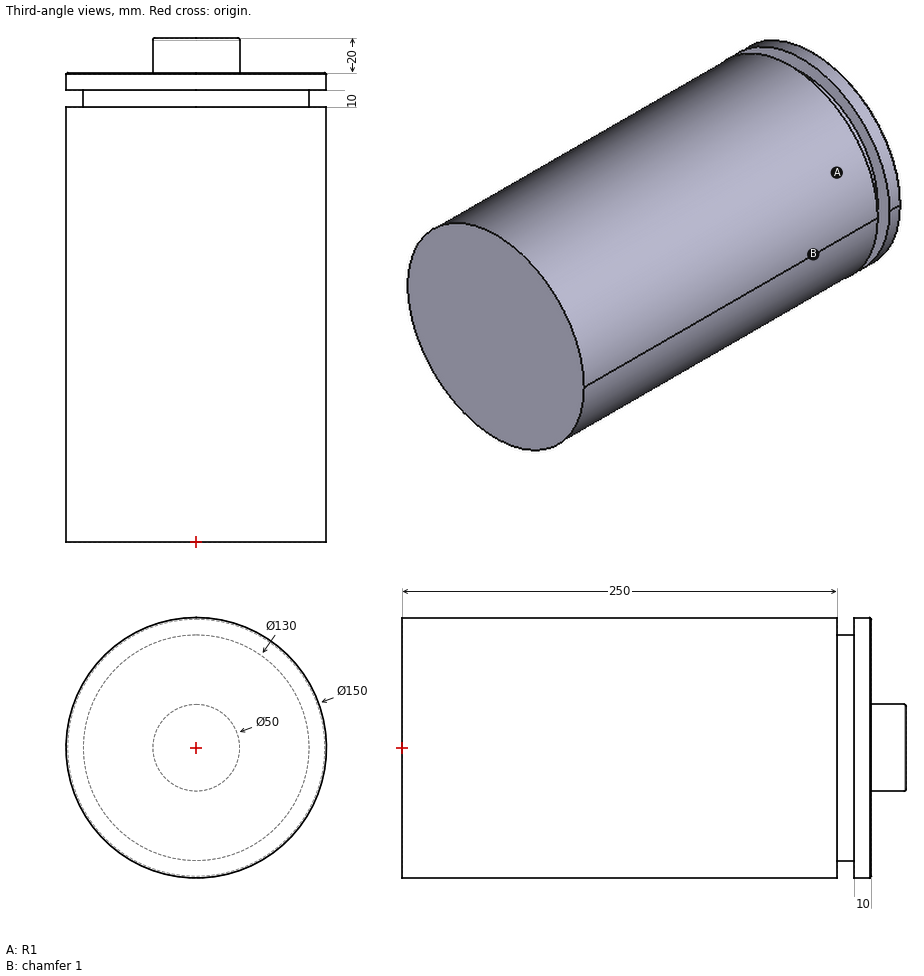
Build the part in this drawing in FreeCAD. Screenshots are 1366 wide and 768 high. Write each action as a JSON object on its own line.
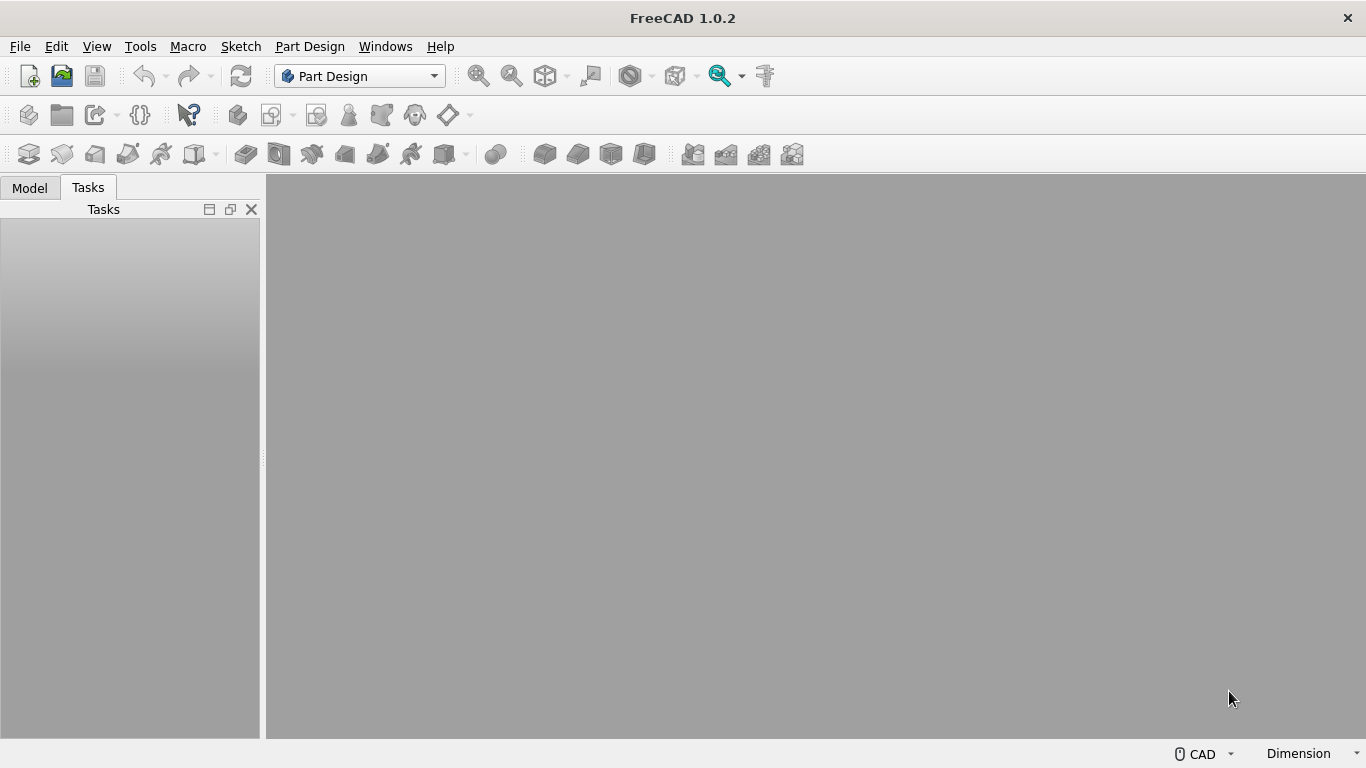
{"action": "key", "text": "ctrl+n"}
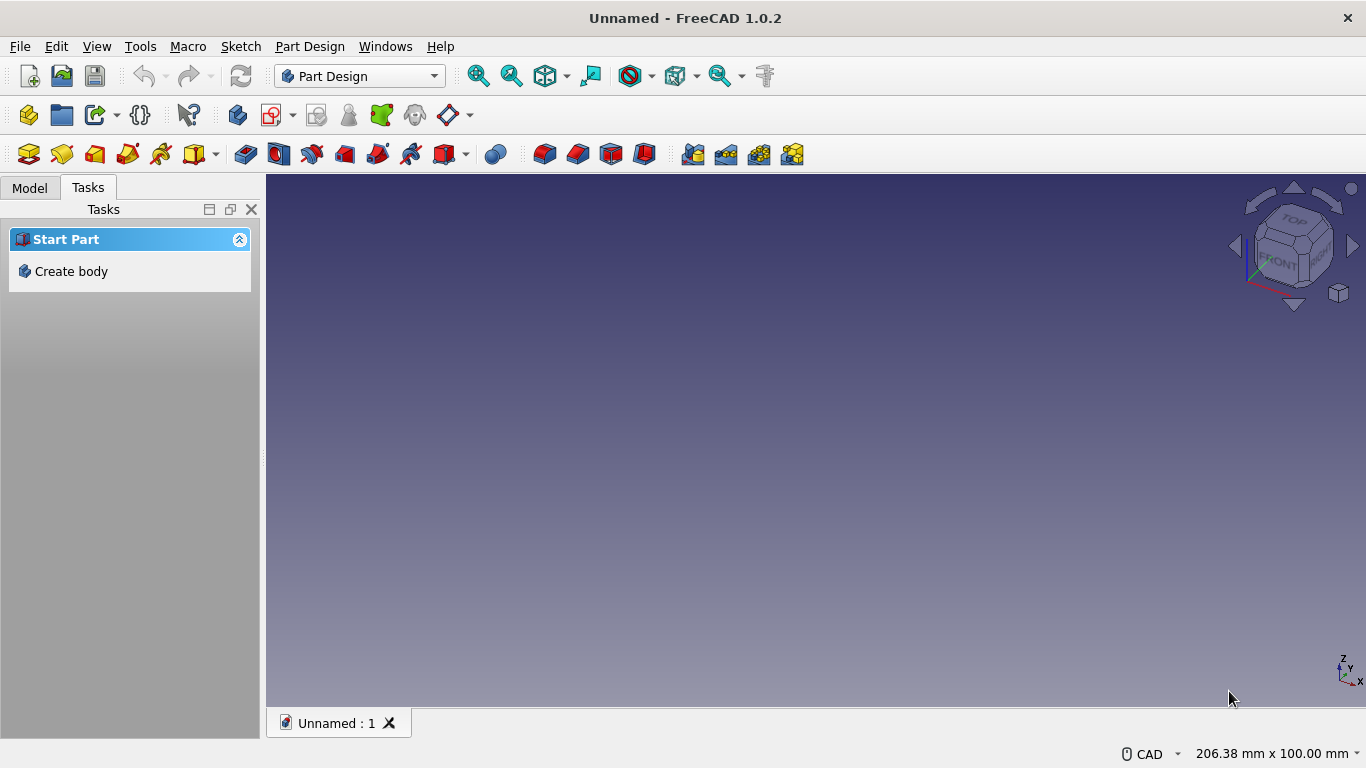
{"action": "left_click", "coordinate": [270, 116]}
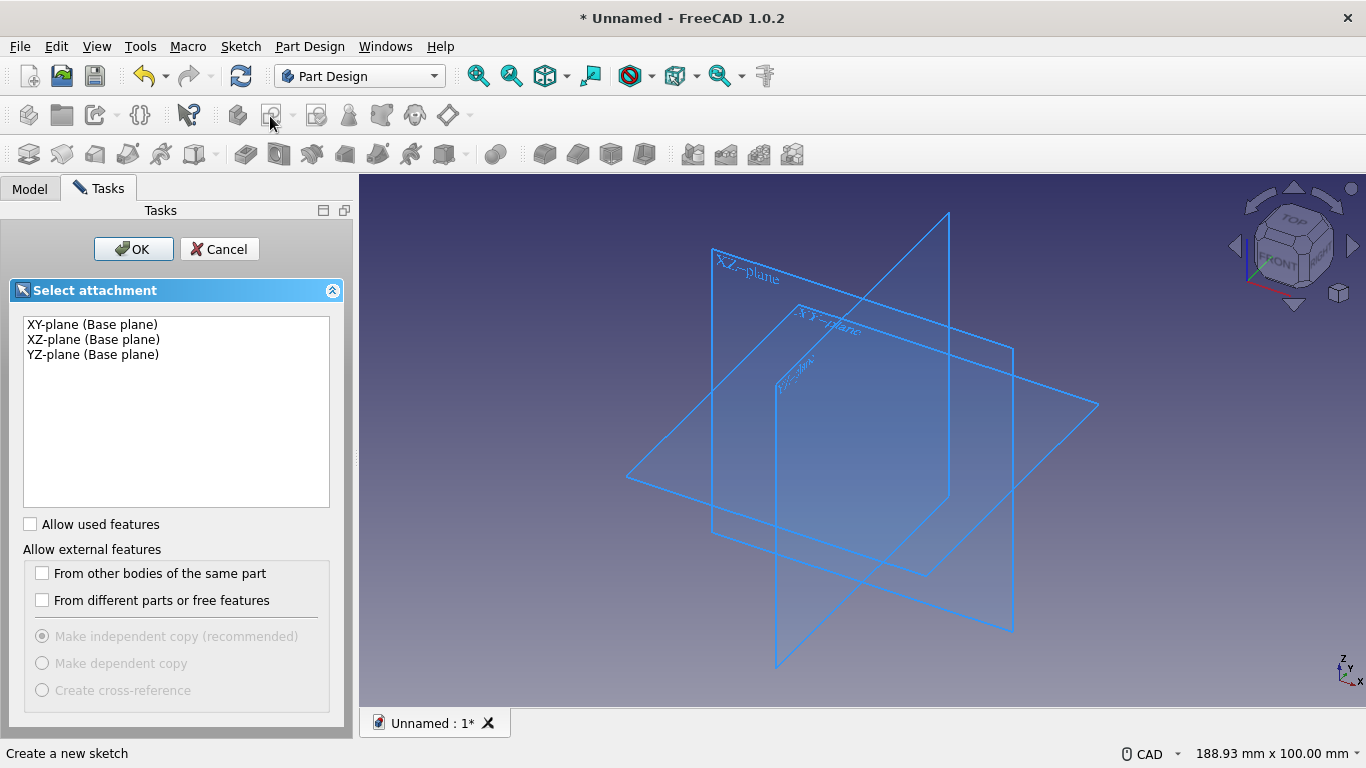
{"action": "left_click", "coordinate": [84, 340]}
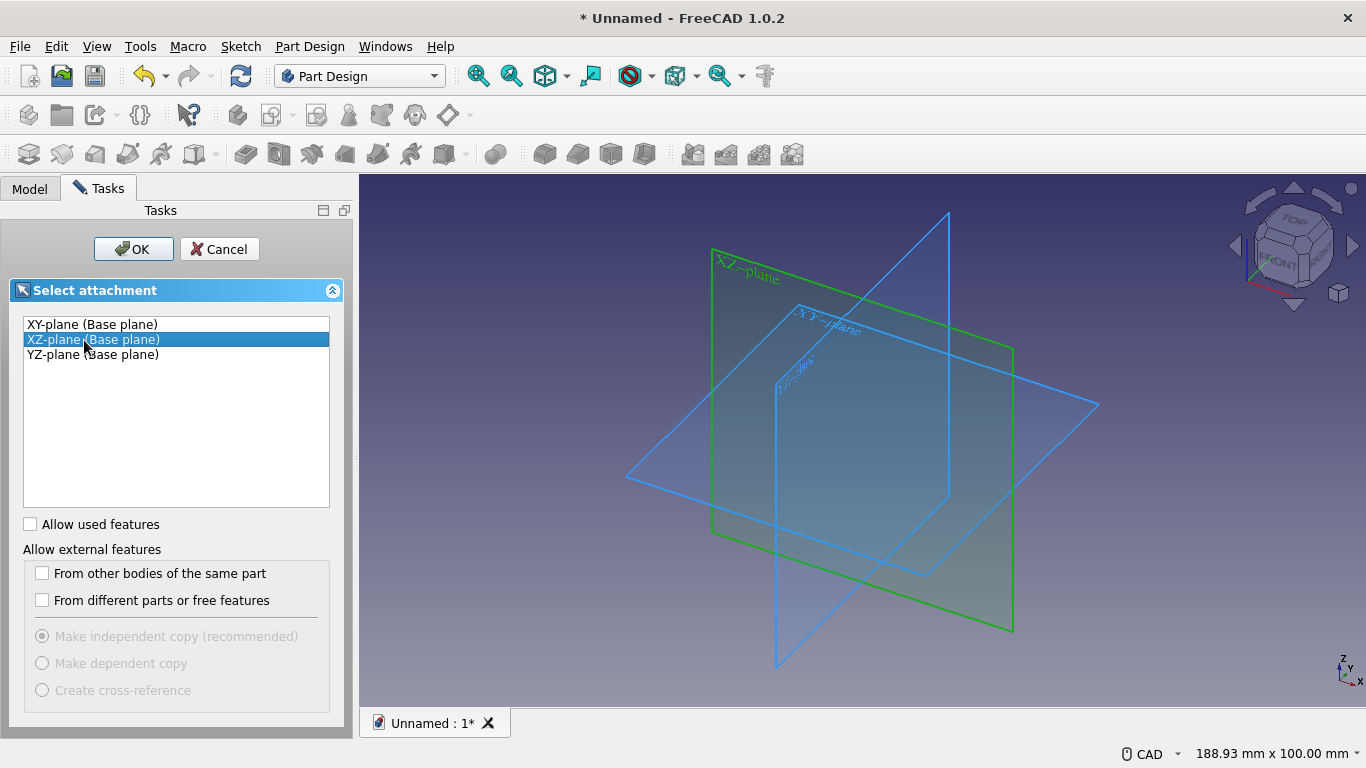
{"action": "left_click", "coordinate": [134, 249]}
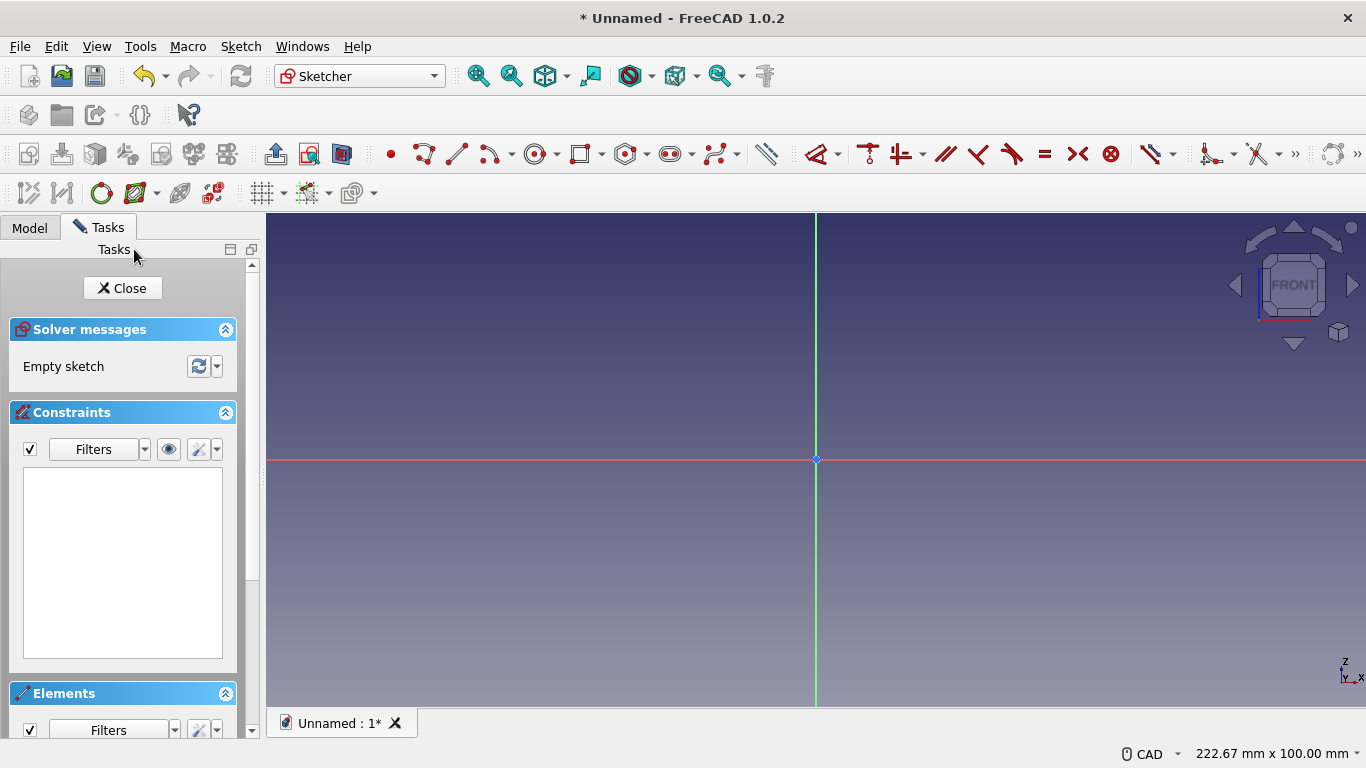
{"action": "scroll", "coordinate": [692, 460], "scroll_direction": "down", "scroll_amount": 4}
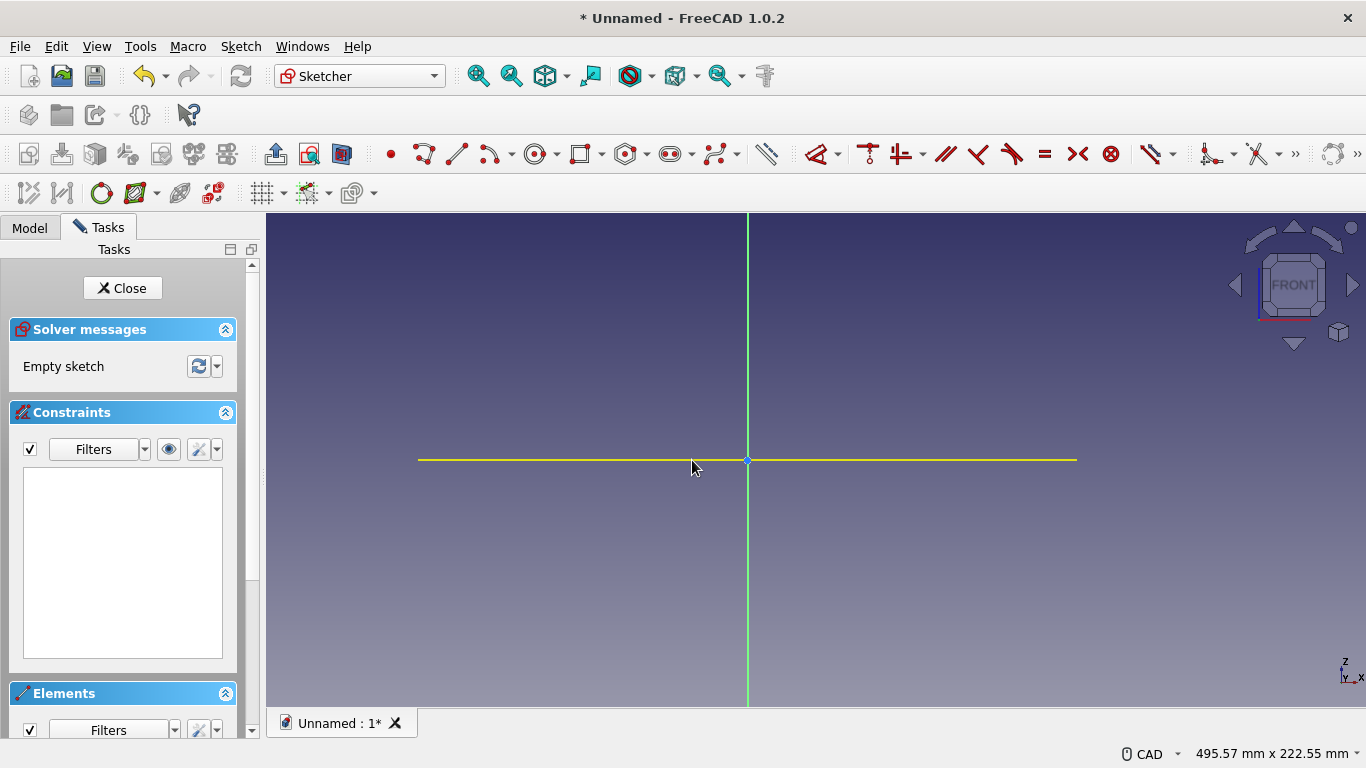
{"action": "left_click", "coordinate": [534, 154]}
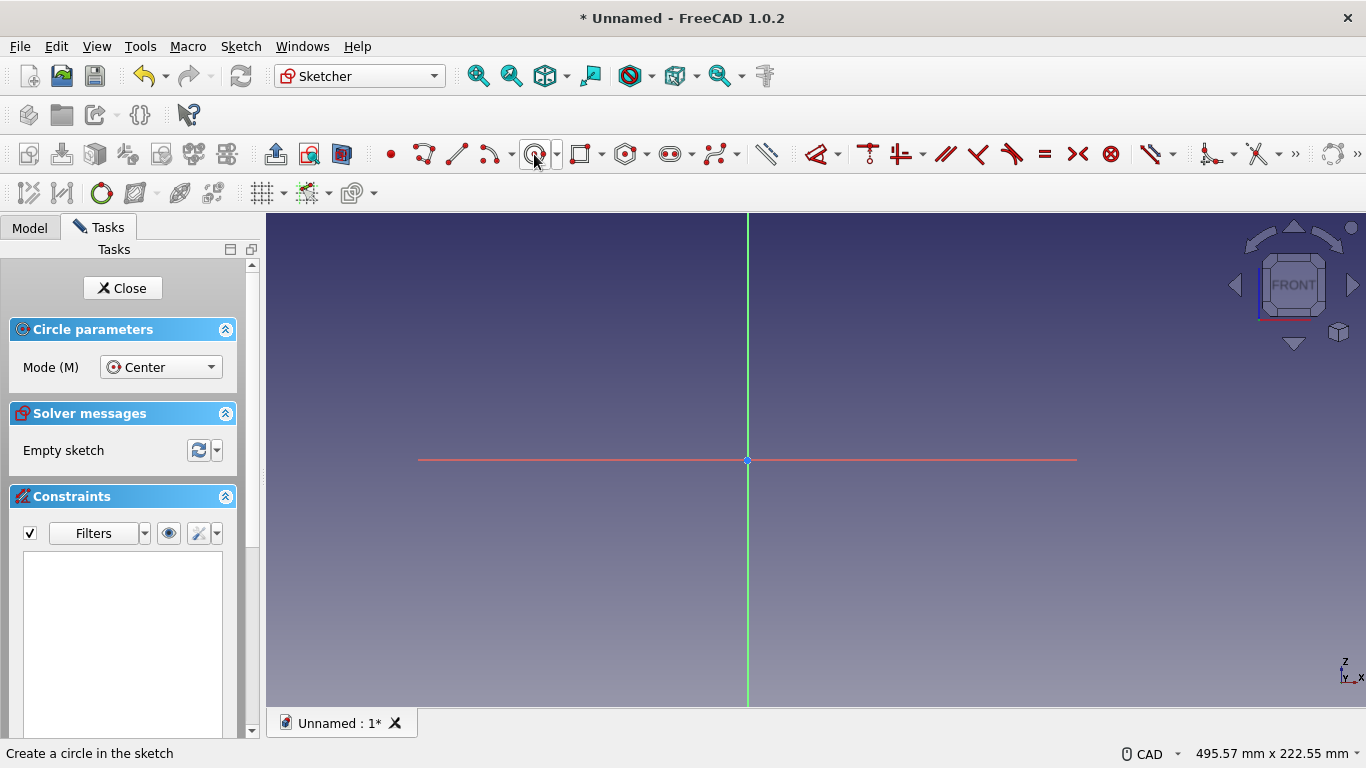
{"action": "left_click", "coordinate": [748, 460]}
{"action": "mouse_move", "coordinate": [866, 343]}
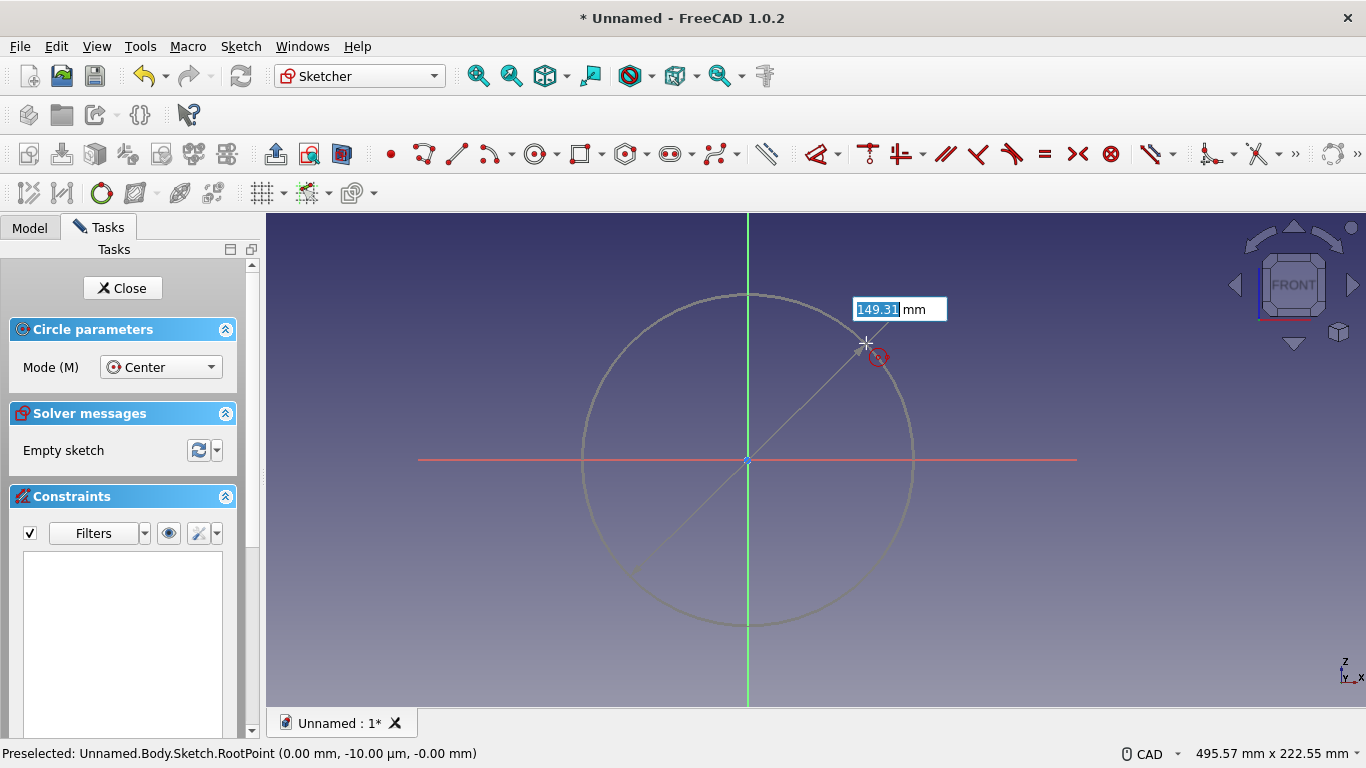
{"action": "type", "text": "150"}
{"action": "key", "text": "Return"}
{"action": "key", "text": "Escape"}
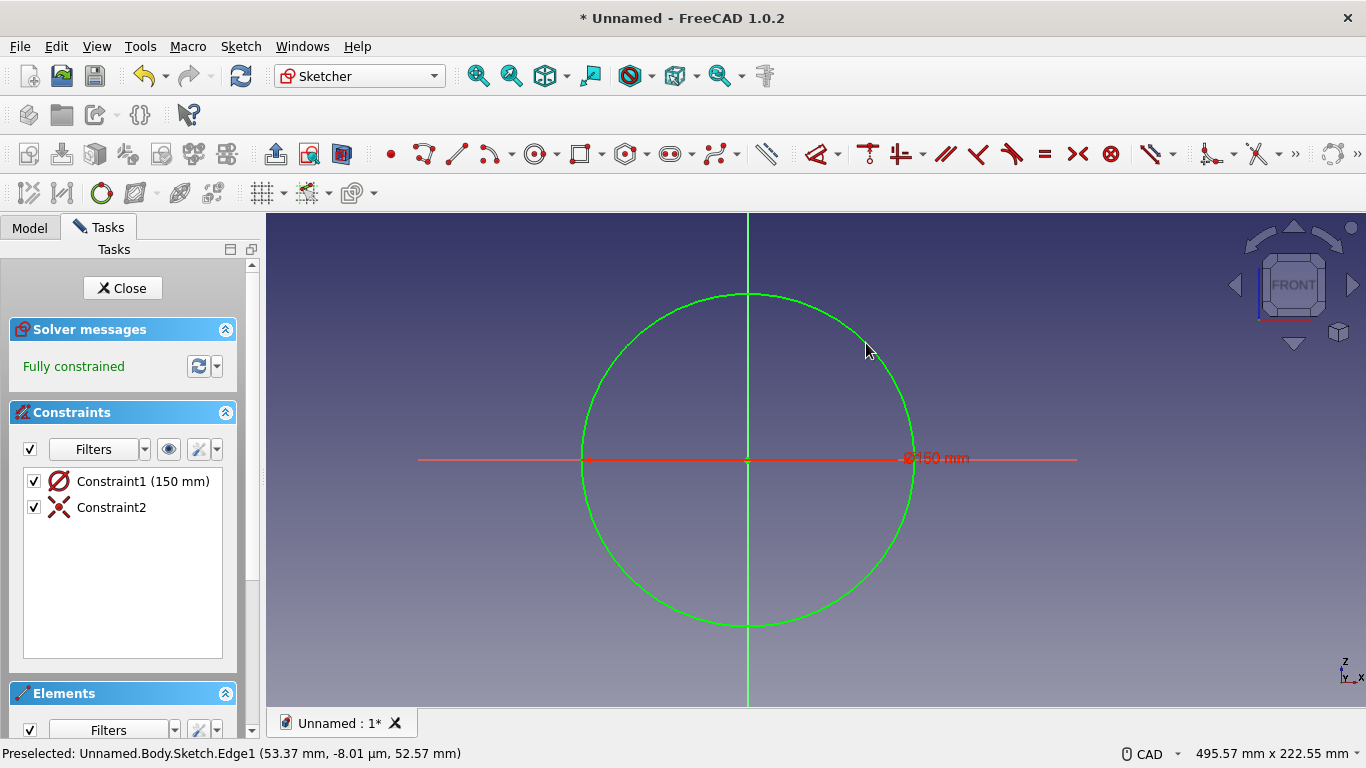
{"action": "left_click", "coordinate": [123, 288]}